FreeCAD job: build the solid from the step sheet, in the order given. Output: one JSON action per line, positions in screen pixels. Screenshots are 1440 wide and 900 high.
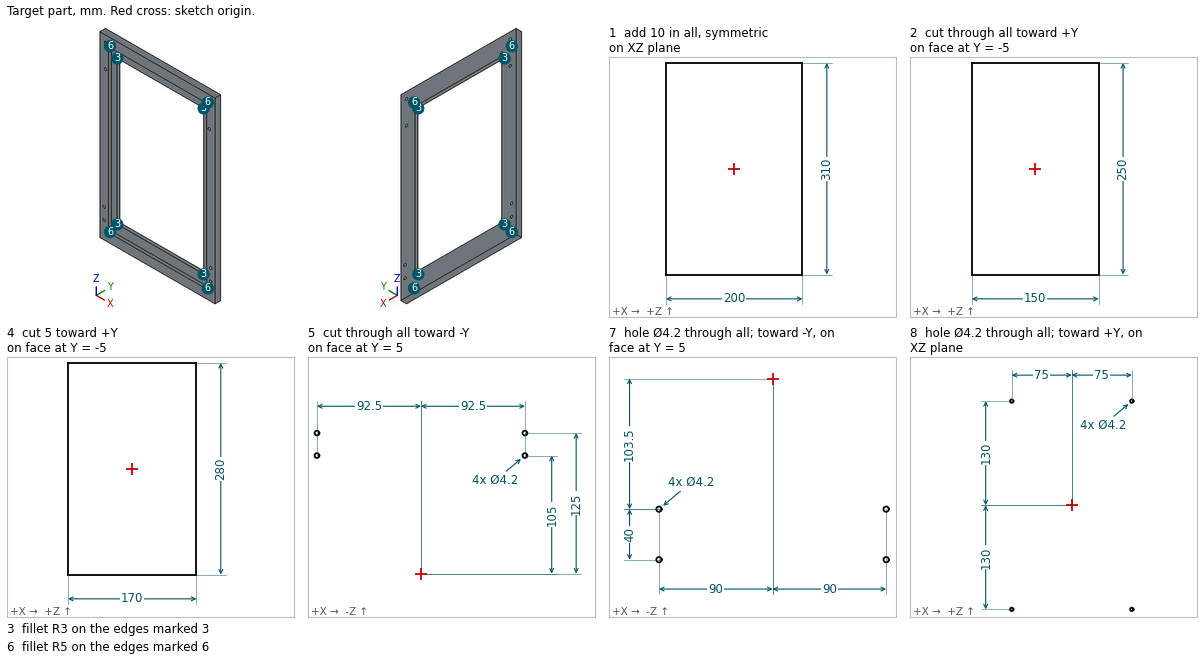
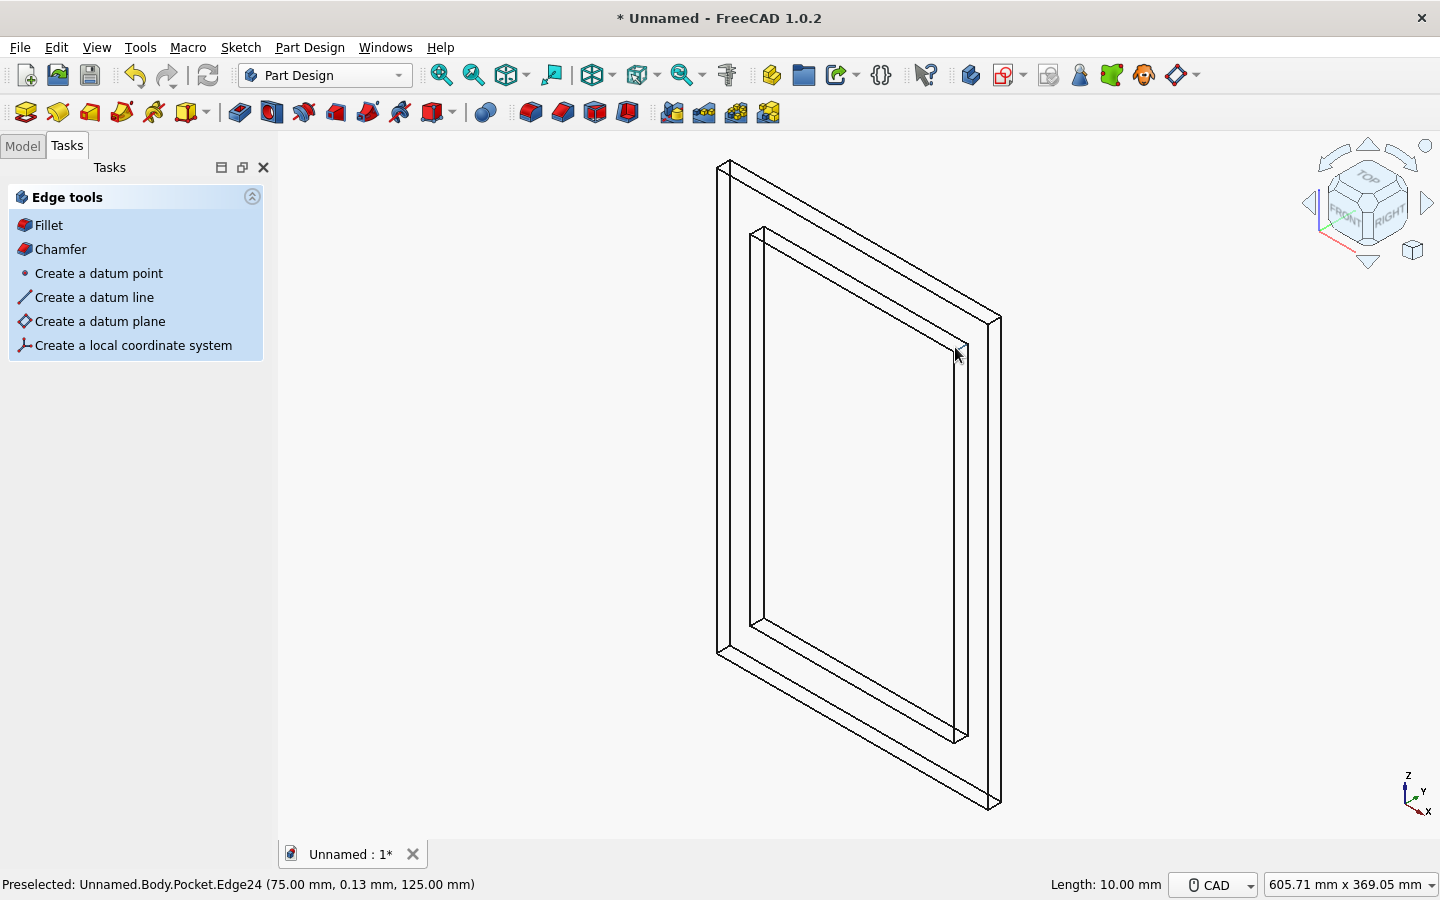
{"action": "left_click", "coordinate": [961, 739], "text": "ctrl"}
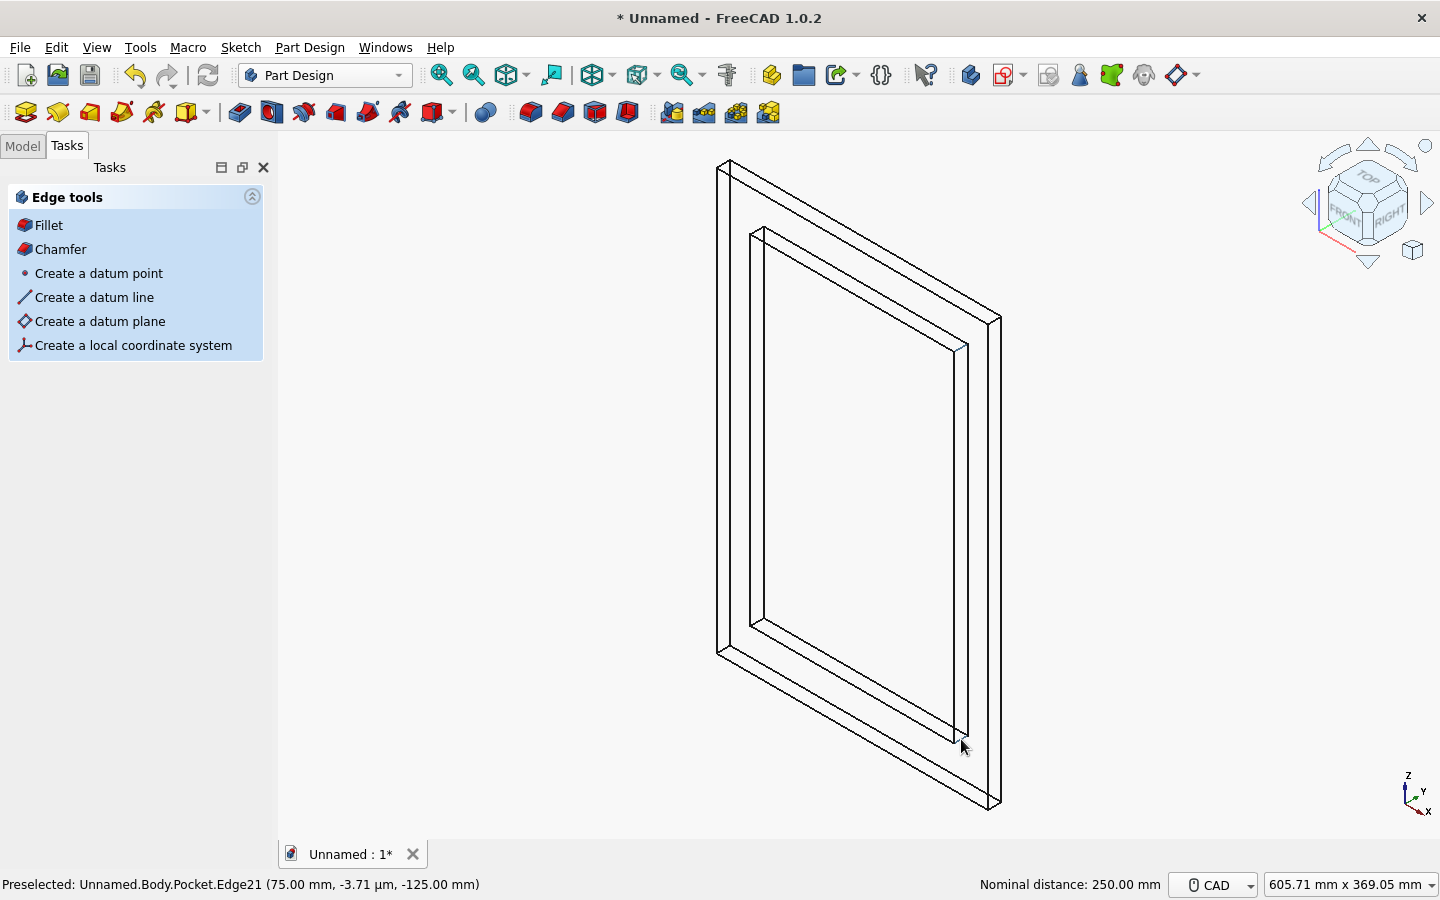
{"action": "left_click", "coordinate": [757, 621], "text": "ctrl"}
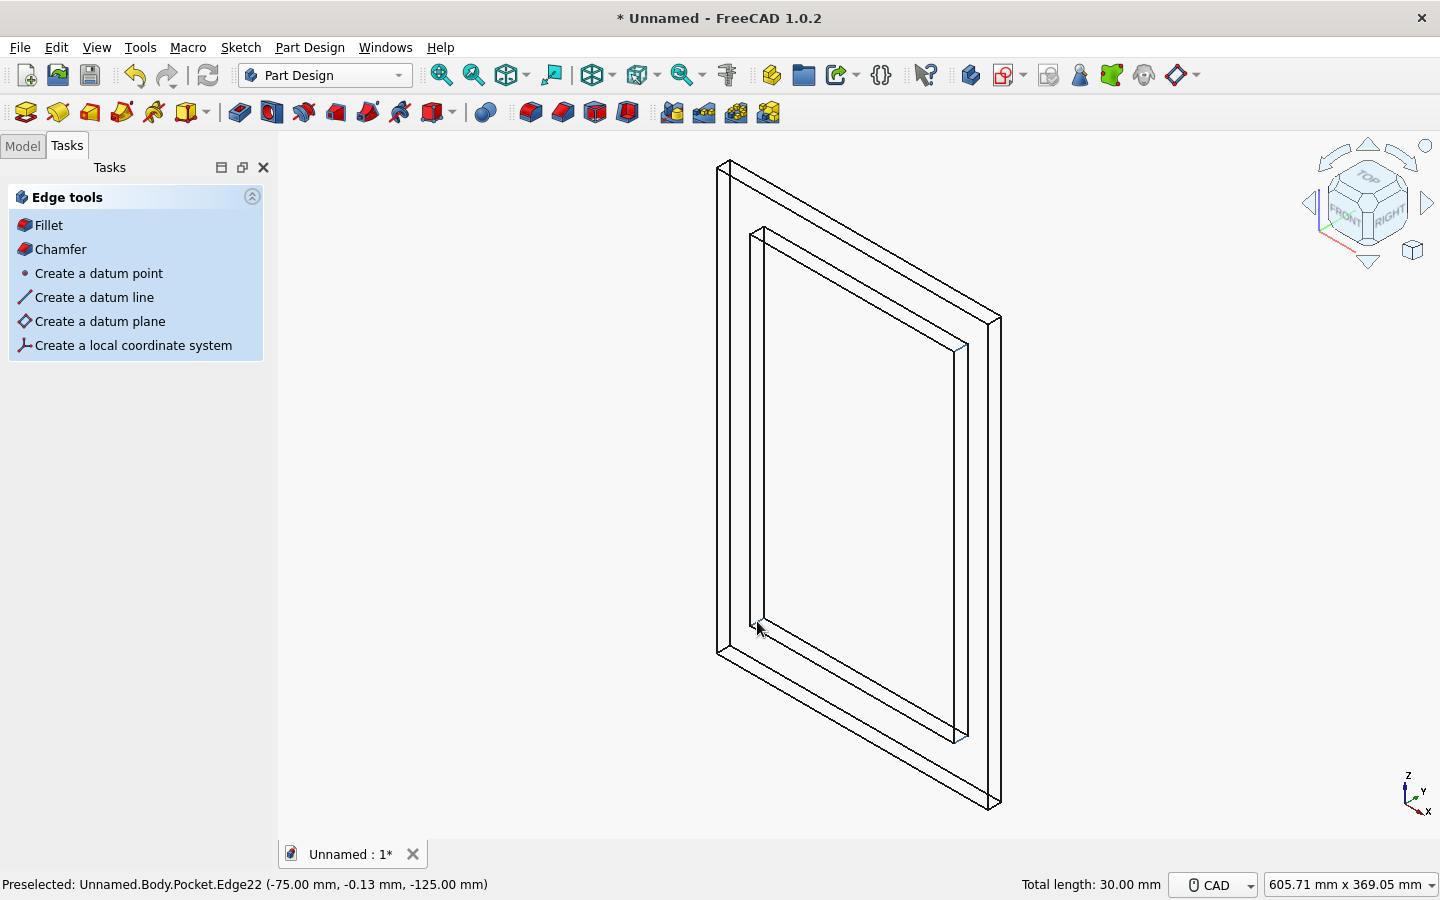
{"action": "left_click", "coordinate": [757, 229], "text": "ctrl"}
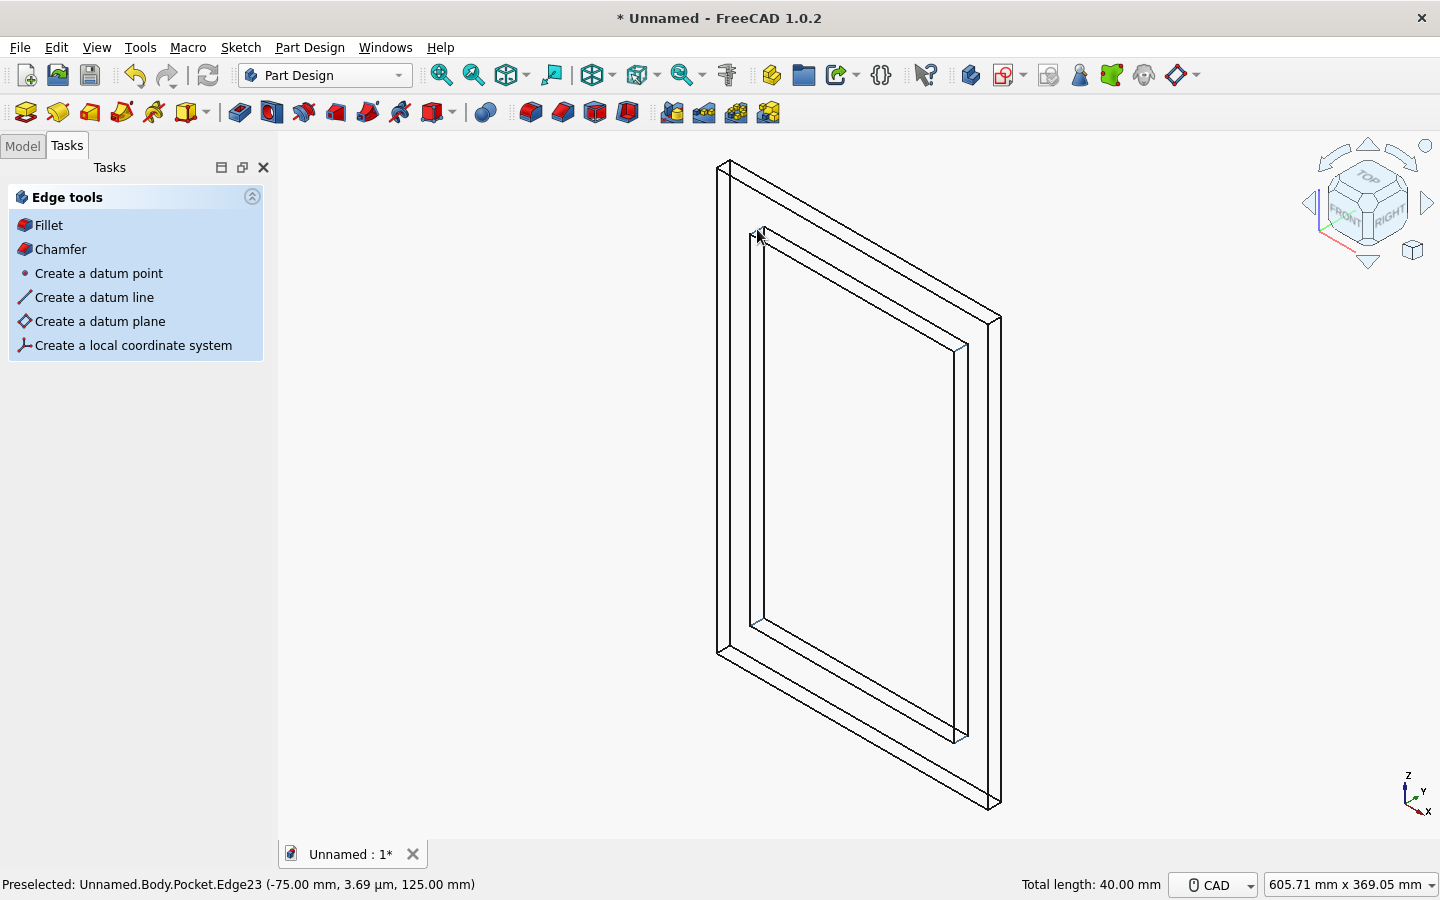
{"action": "key", "text": "v 1"}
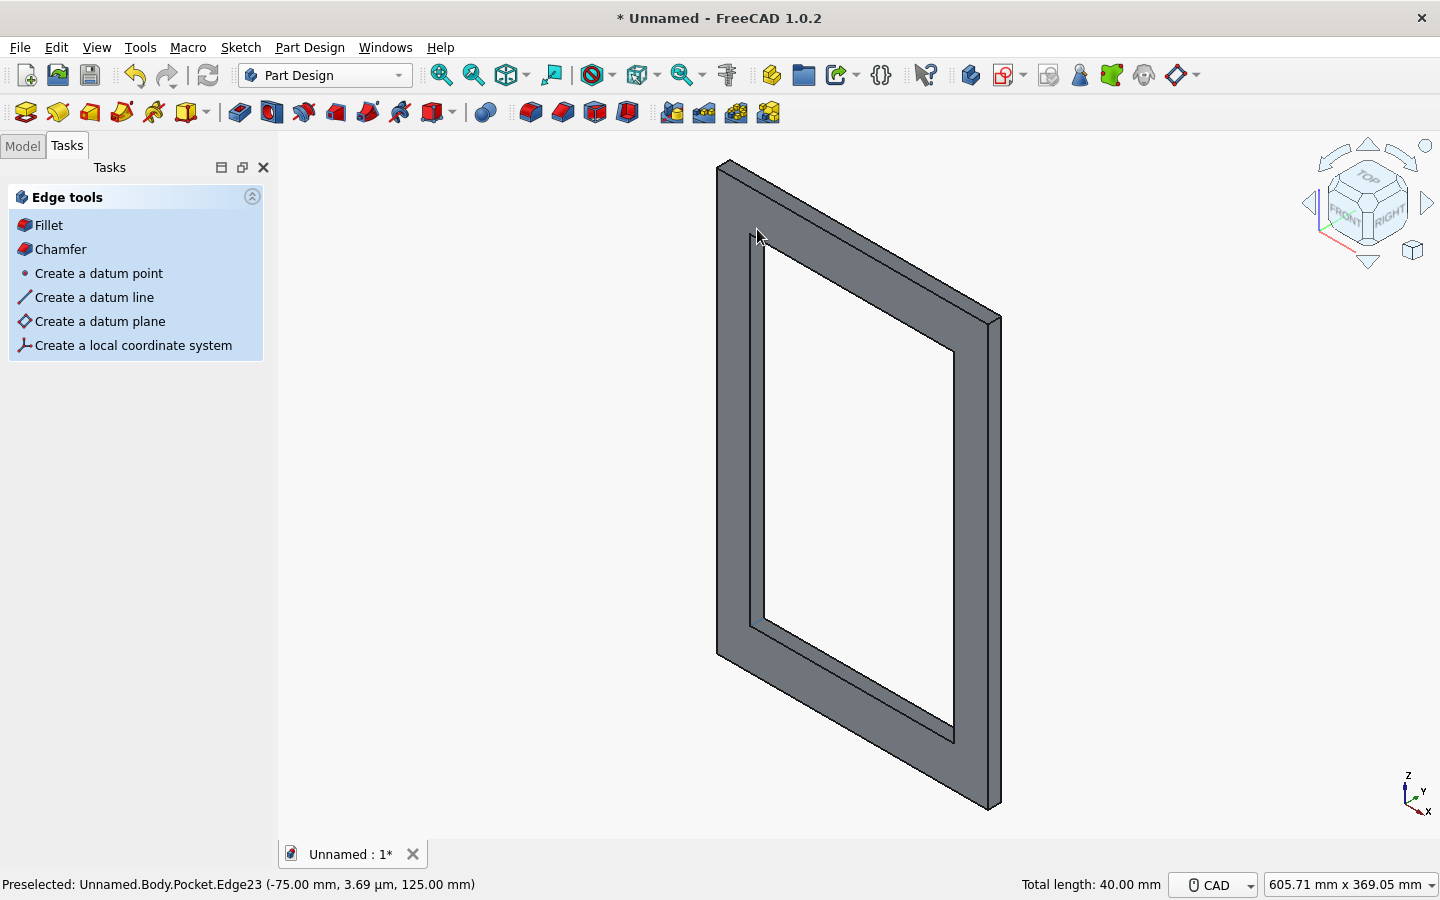
{"action": "left_click", "coordinate": [532, 112]}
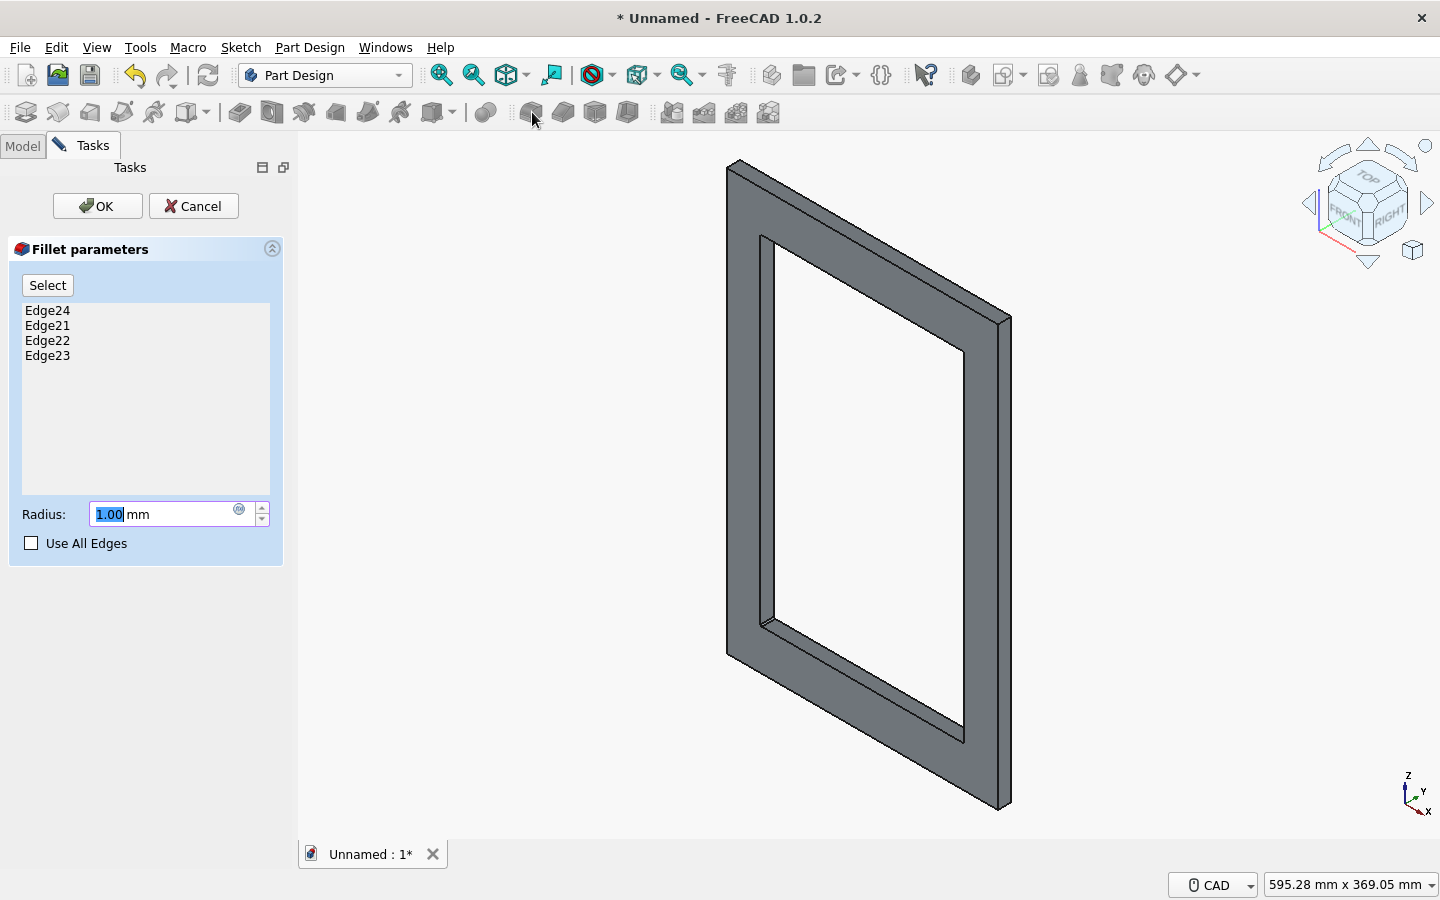
{"action": "type", "text": "3"}
{"action": "key", "text": "Tab"}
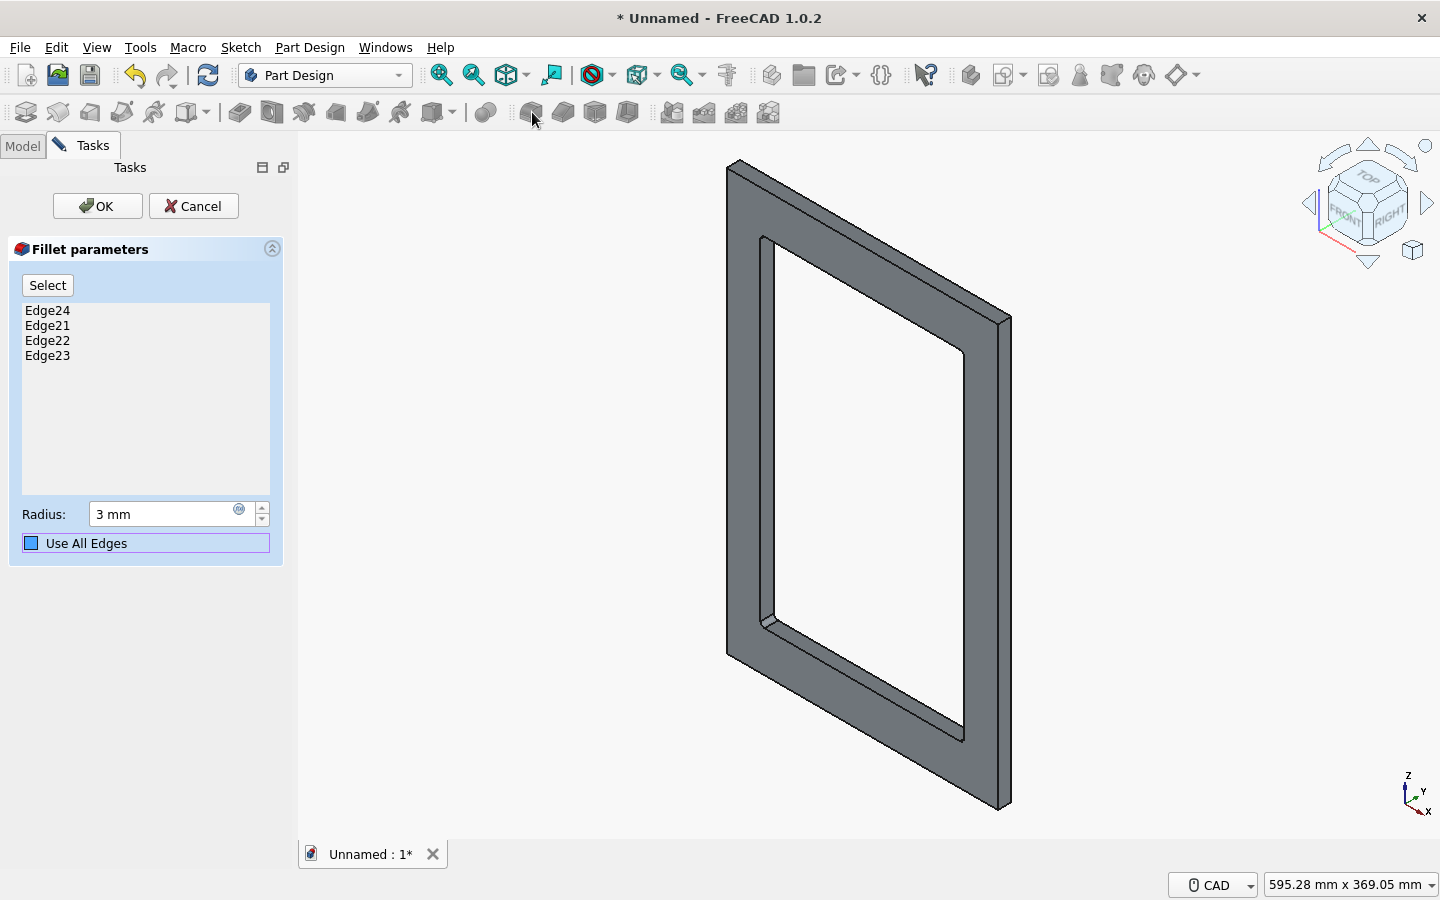
{"action": "left_click", "coordinate": [98, 206]}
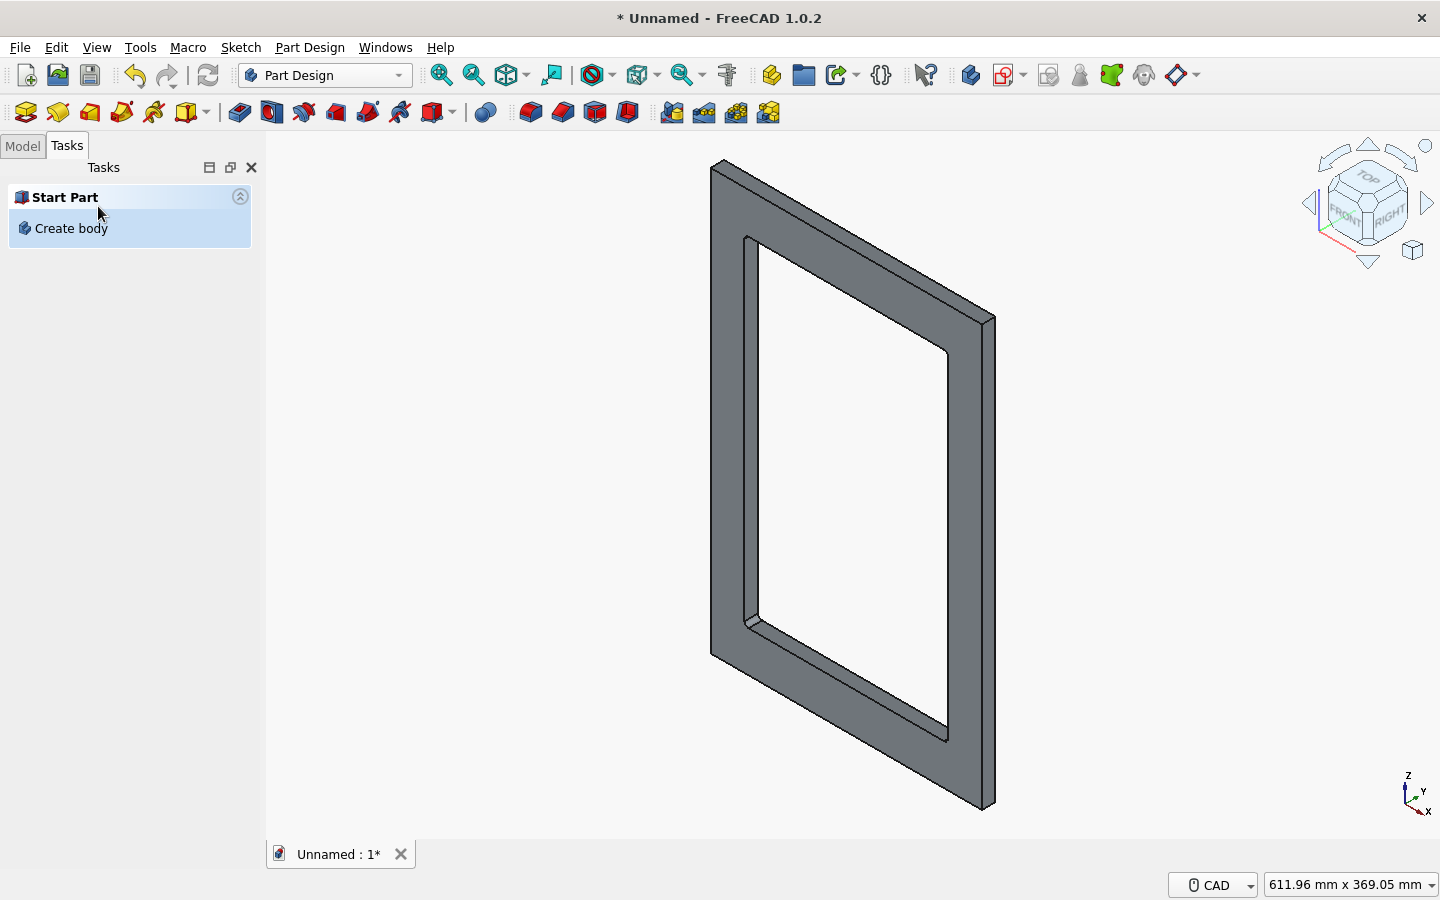
{"action": "left_click", "coordinate": [730, 213]}